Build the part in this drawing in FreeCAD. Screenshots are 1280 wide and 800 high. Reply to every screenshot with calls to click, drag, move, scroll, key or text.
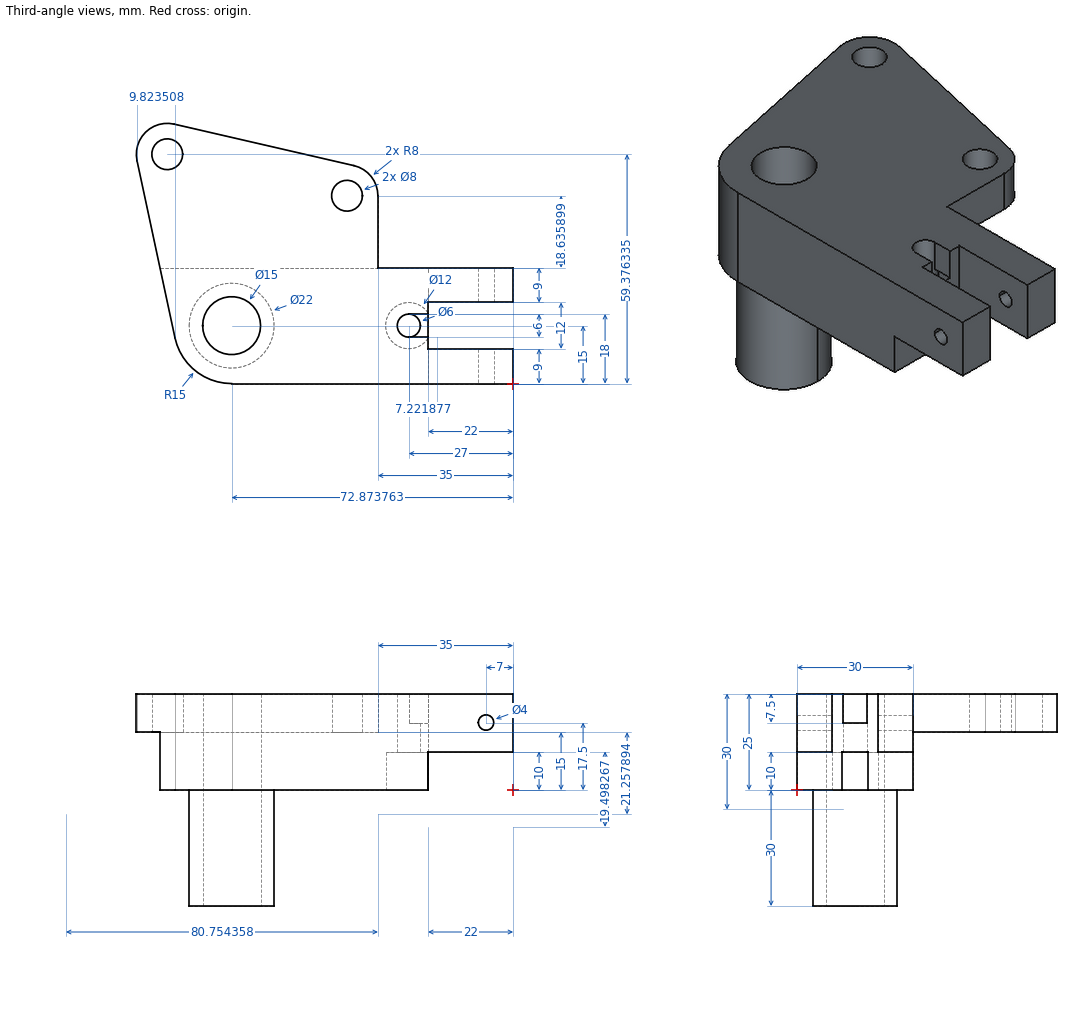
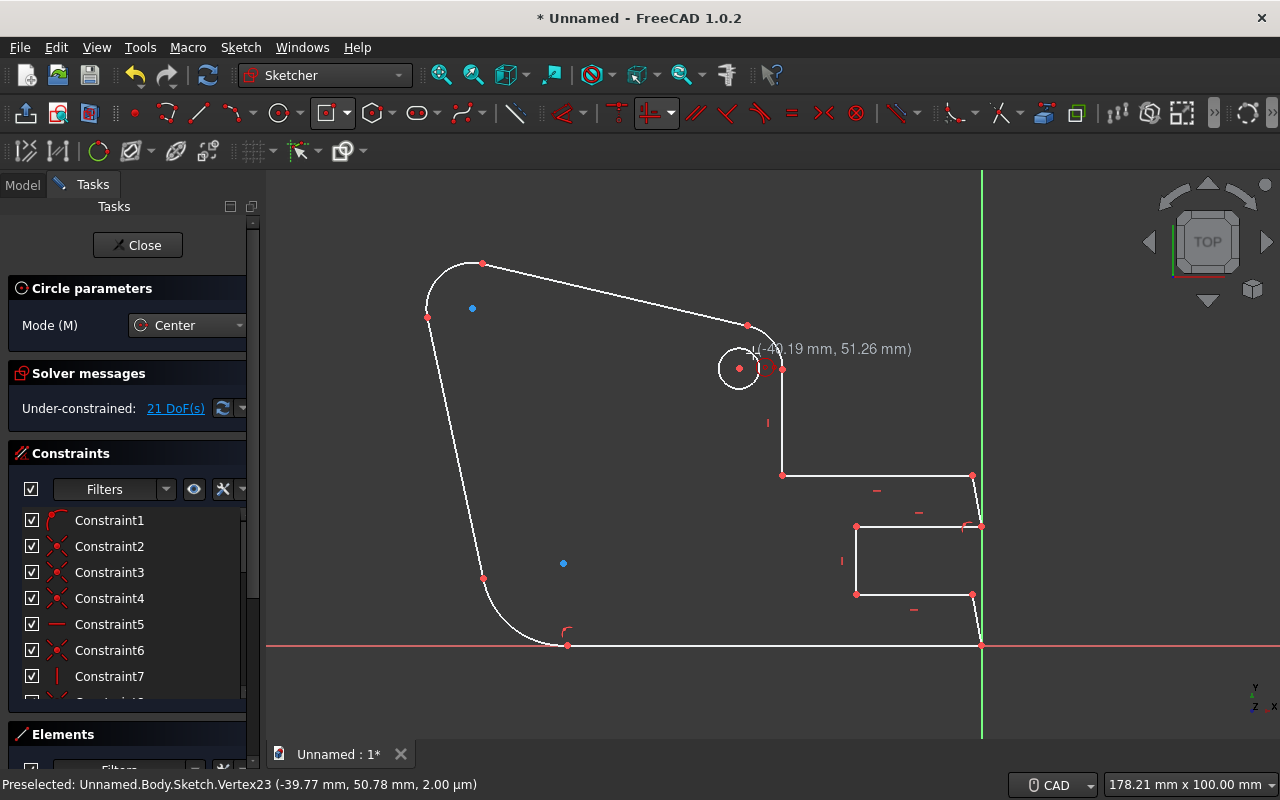
click(472, 308)
click(488, 292)
key(Escape)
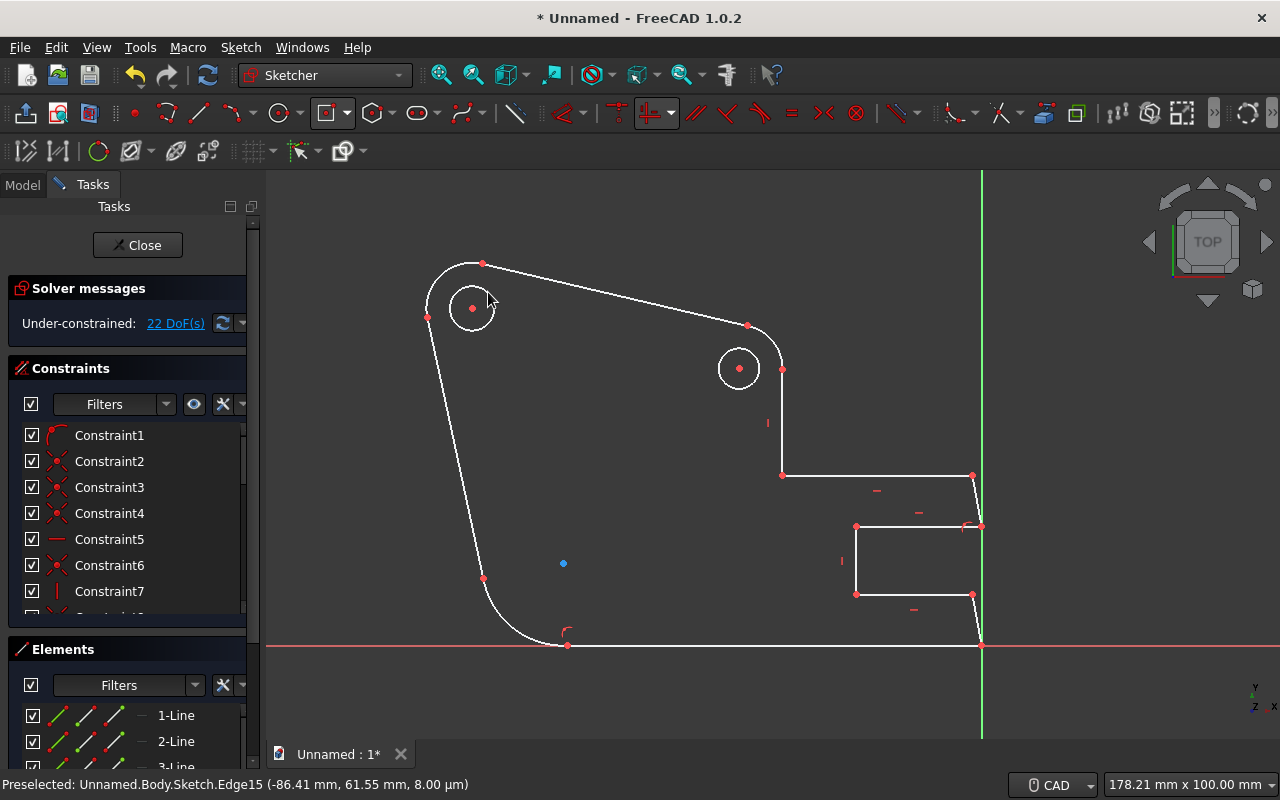
click(692, 646)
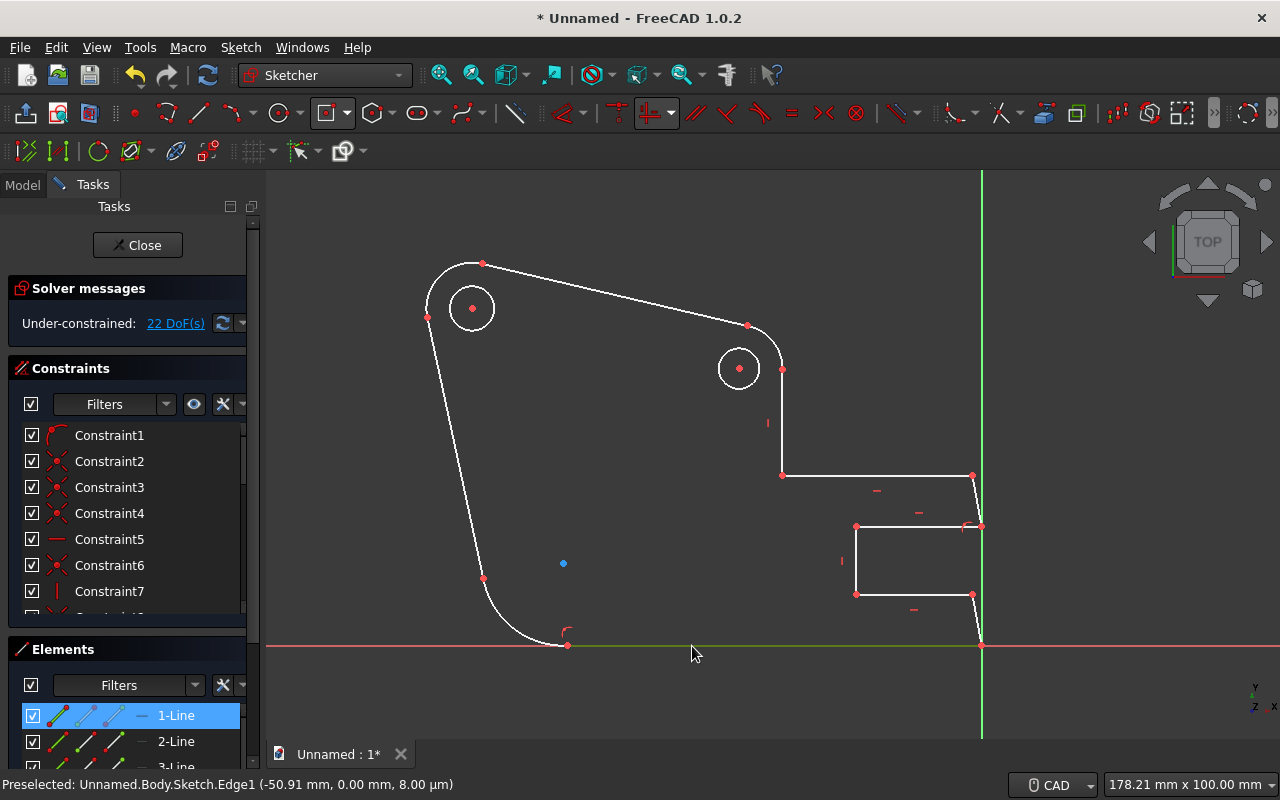
click(497, 611)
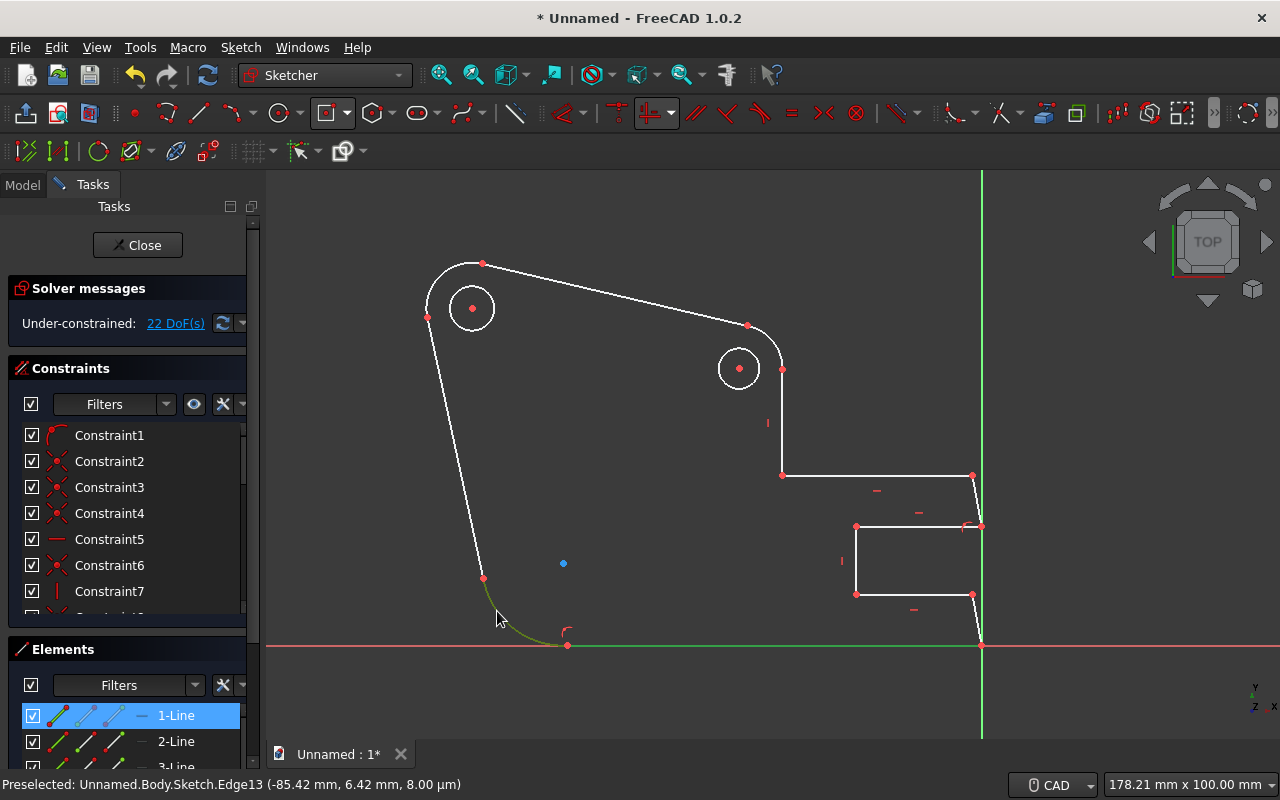
click(760, 114)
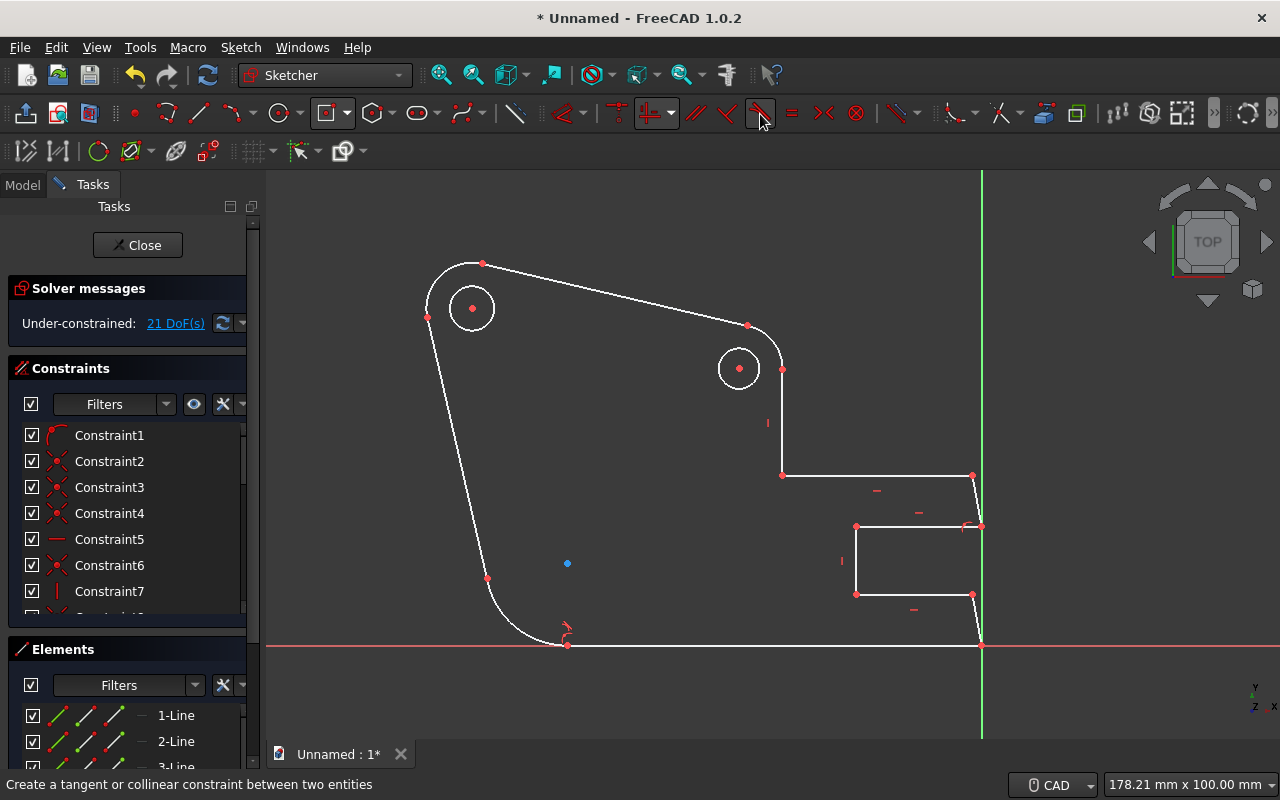
click(782, 444)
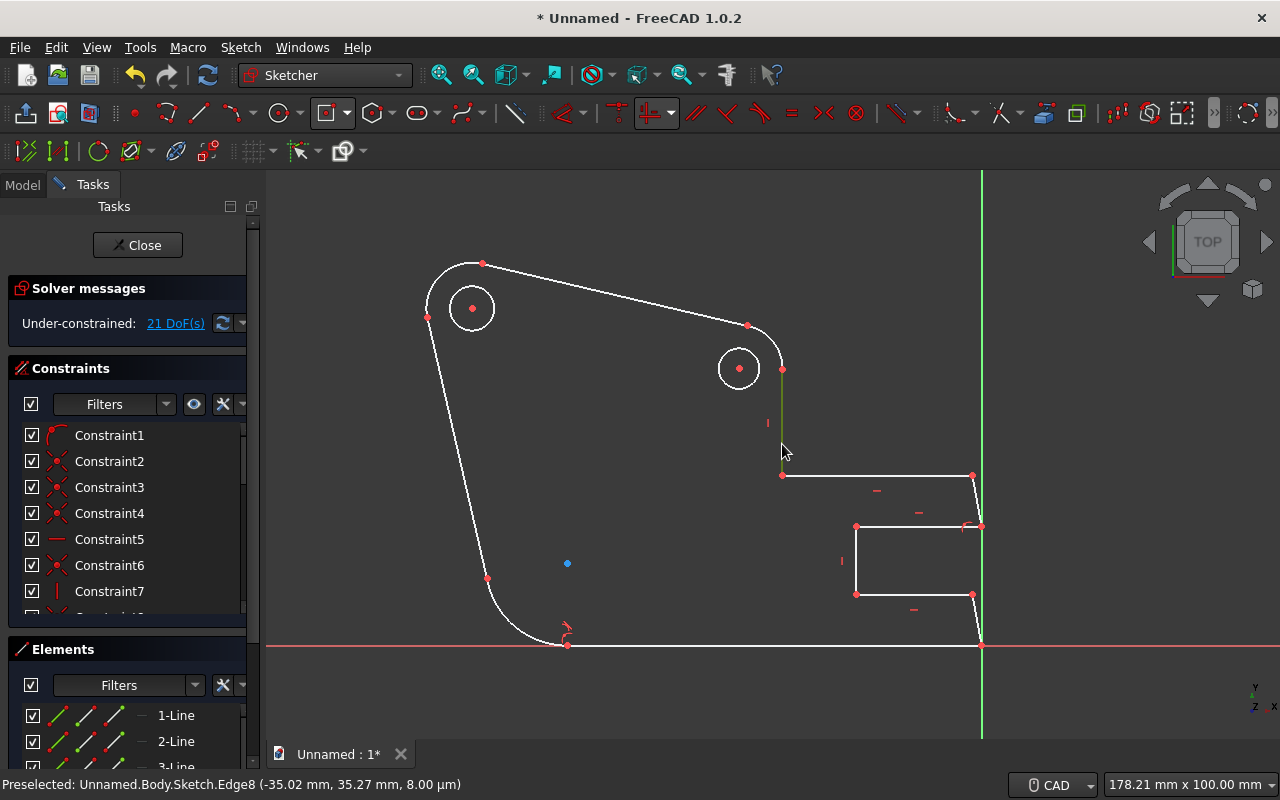
click(779, 352)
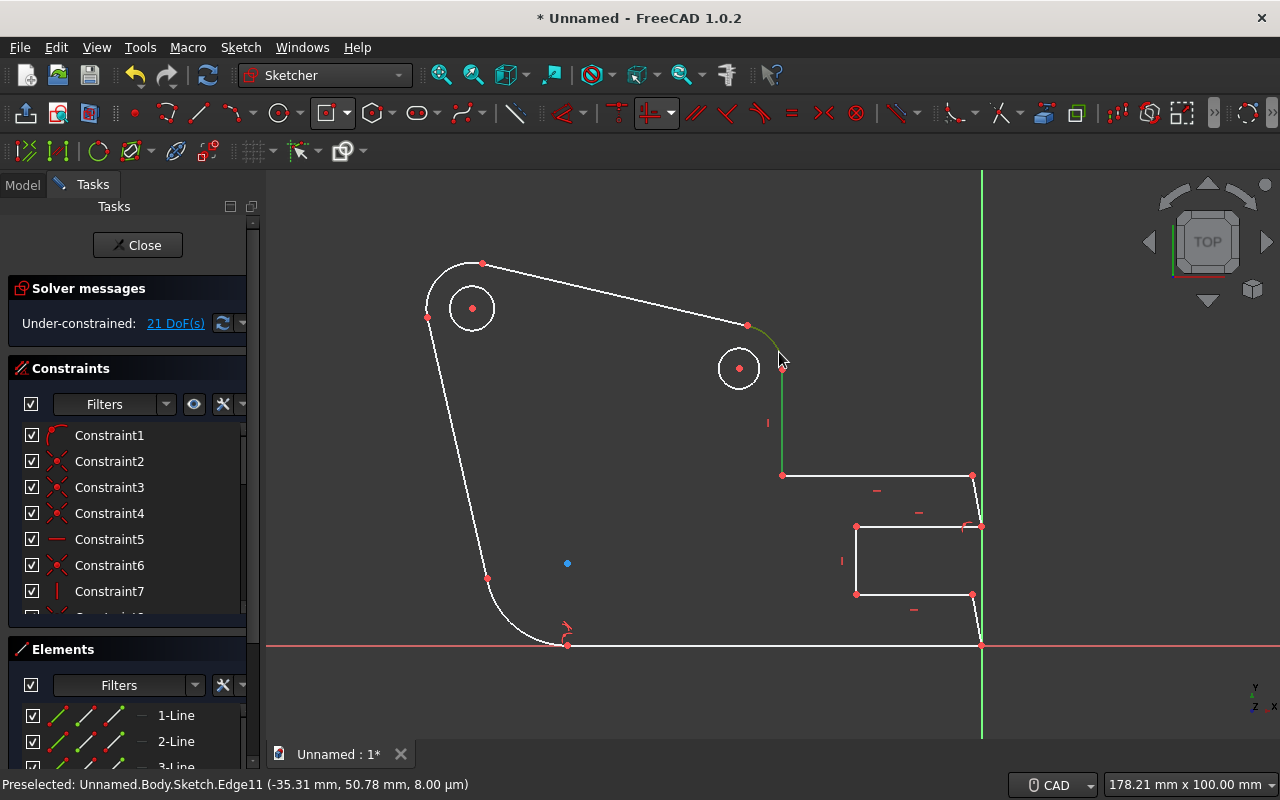
click(760, 114)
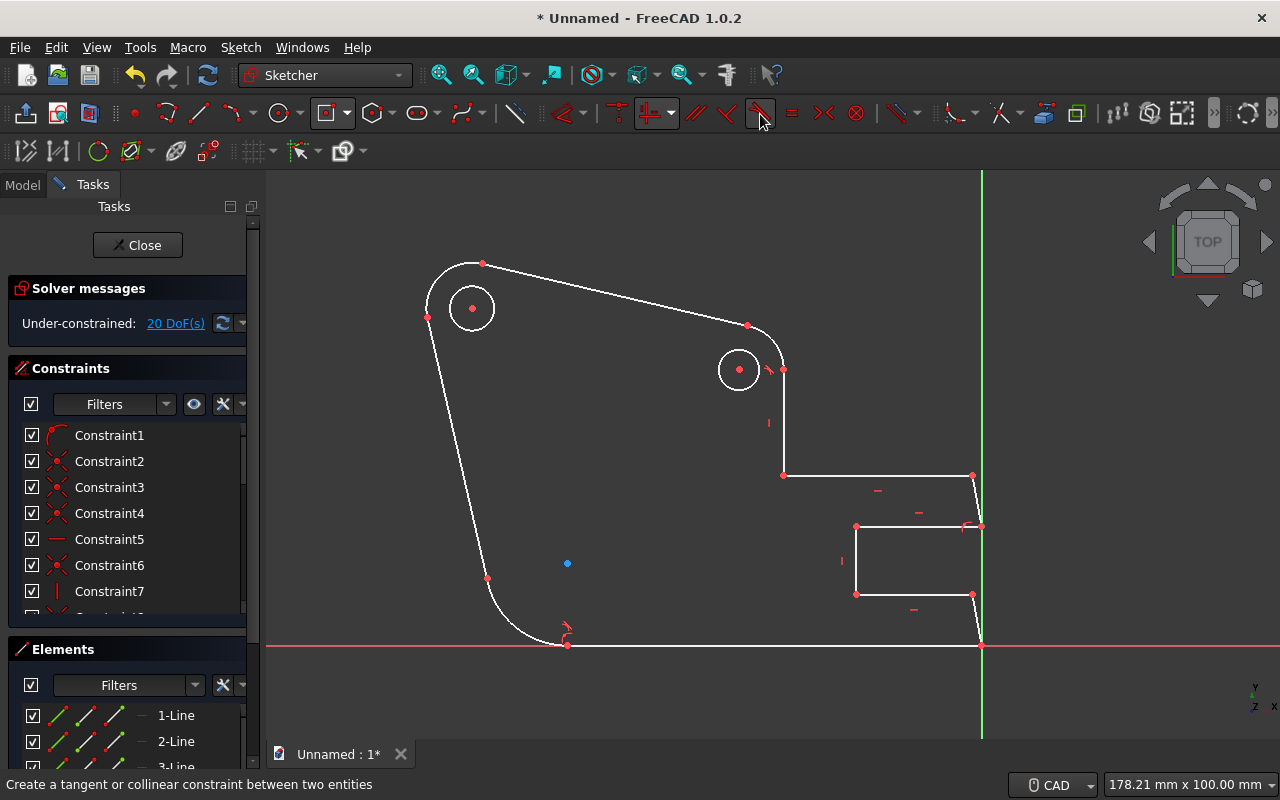
click(668, 307)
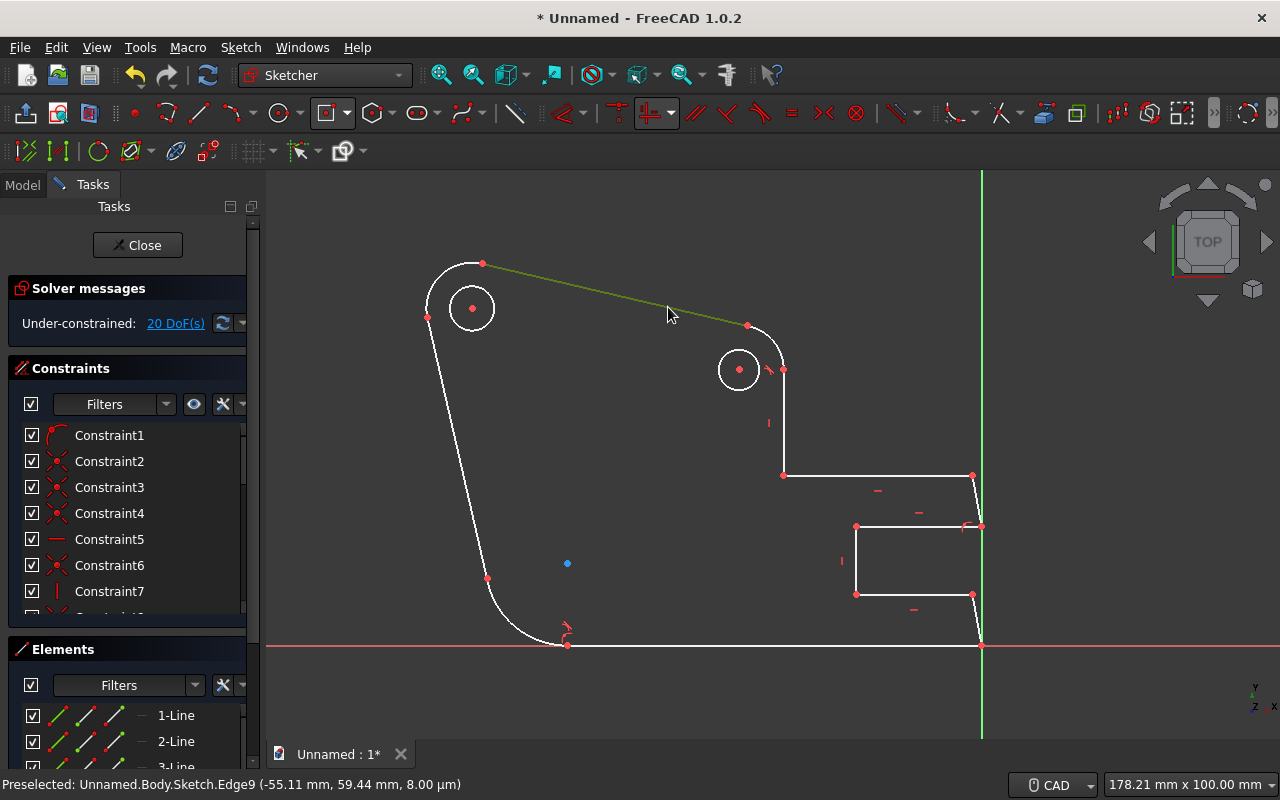
click(780, 352)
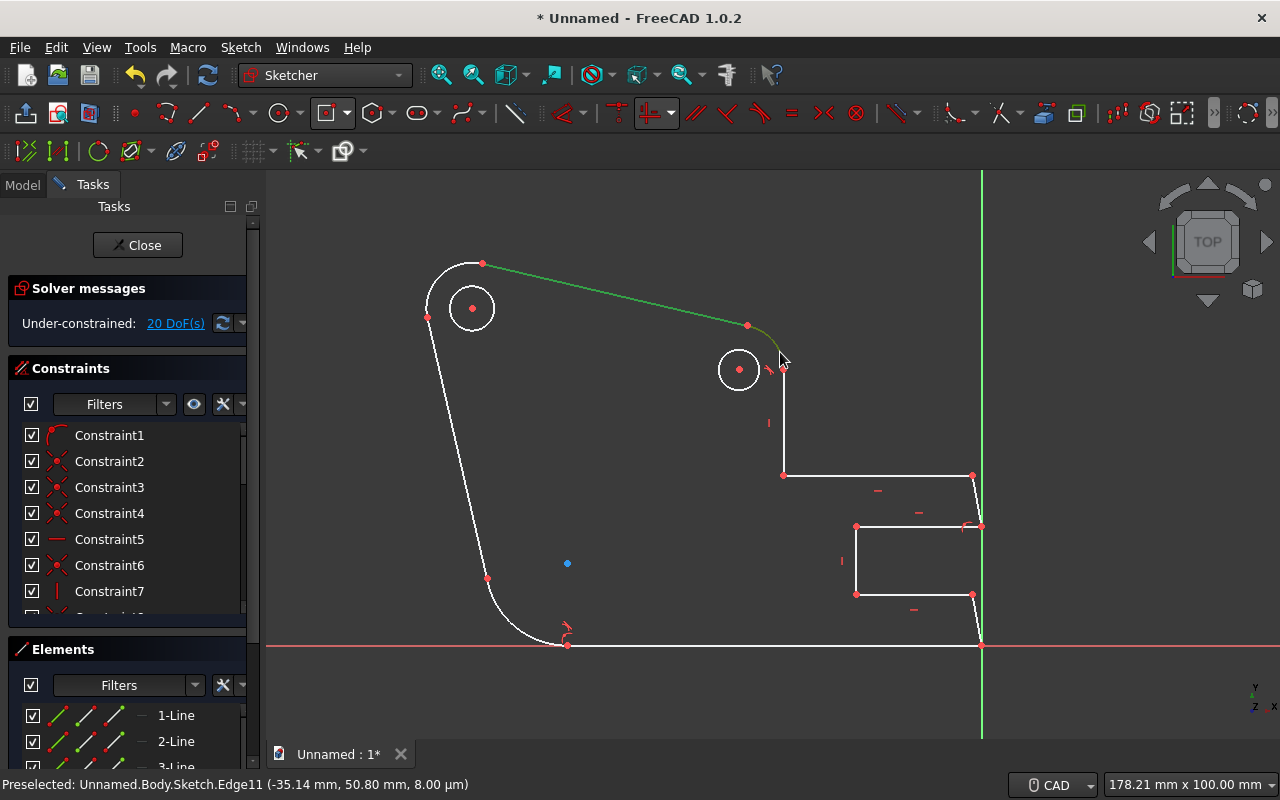
click(760, 114)